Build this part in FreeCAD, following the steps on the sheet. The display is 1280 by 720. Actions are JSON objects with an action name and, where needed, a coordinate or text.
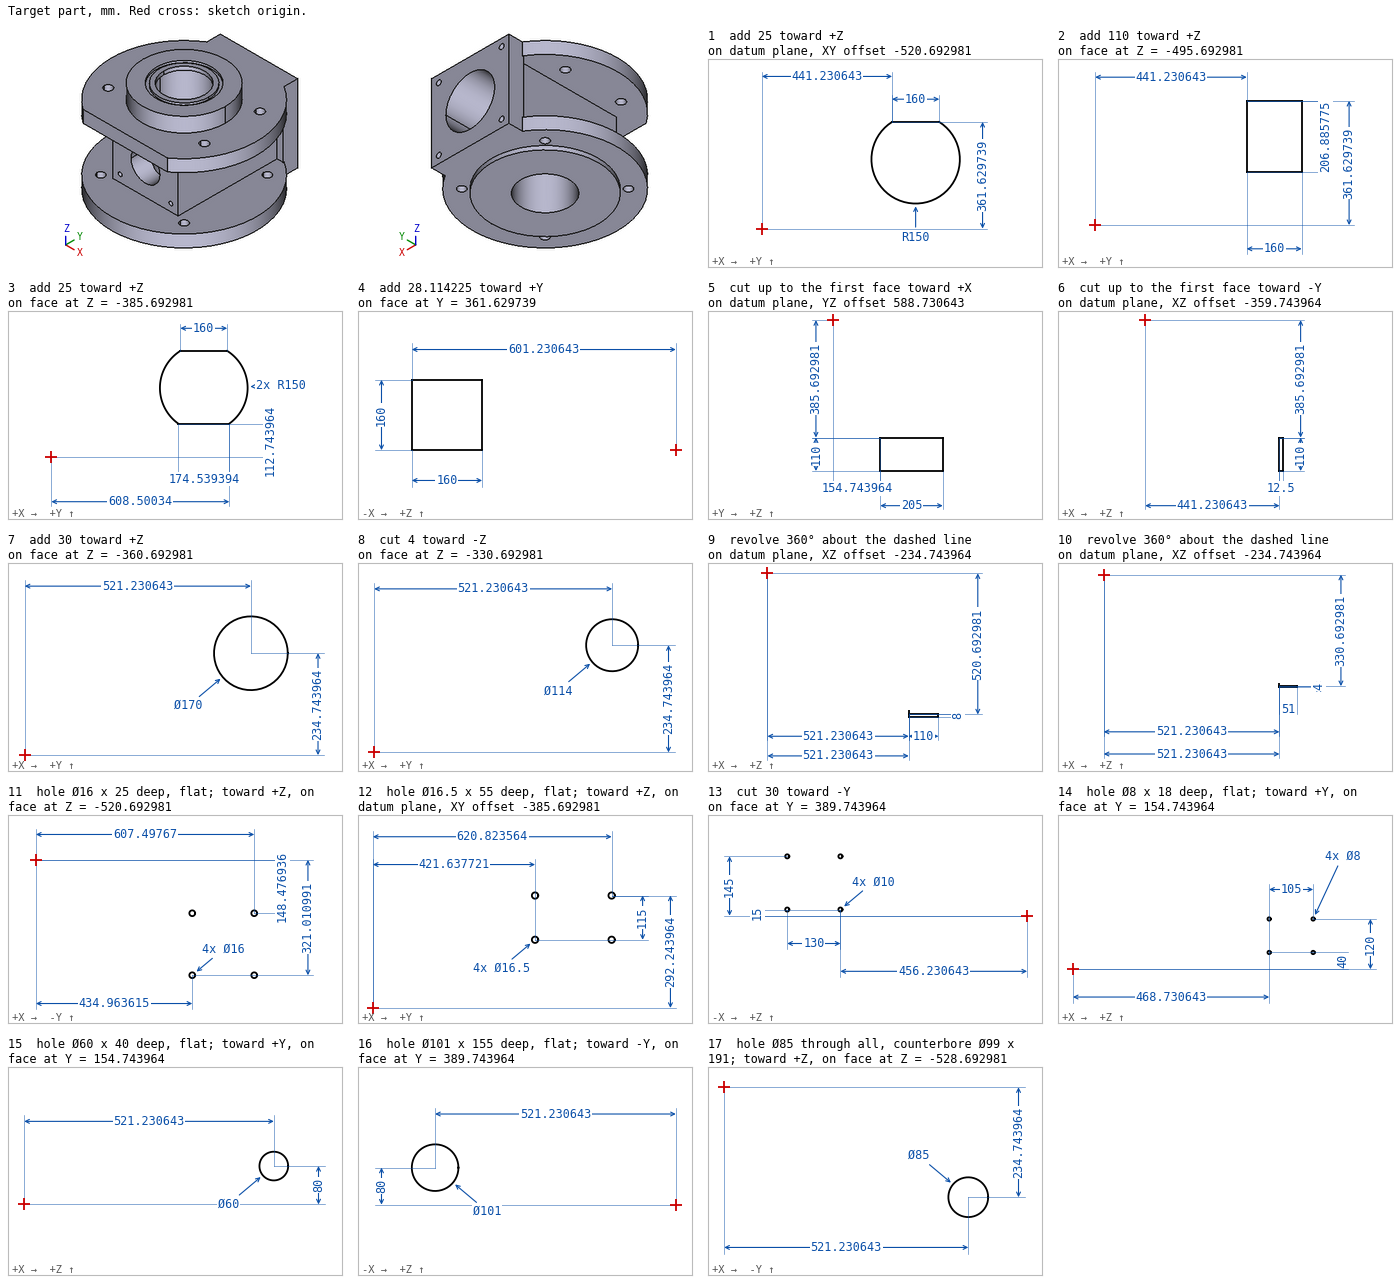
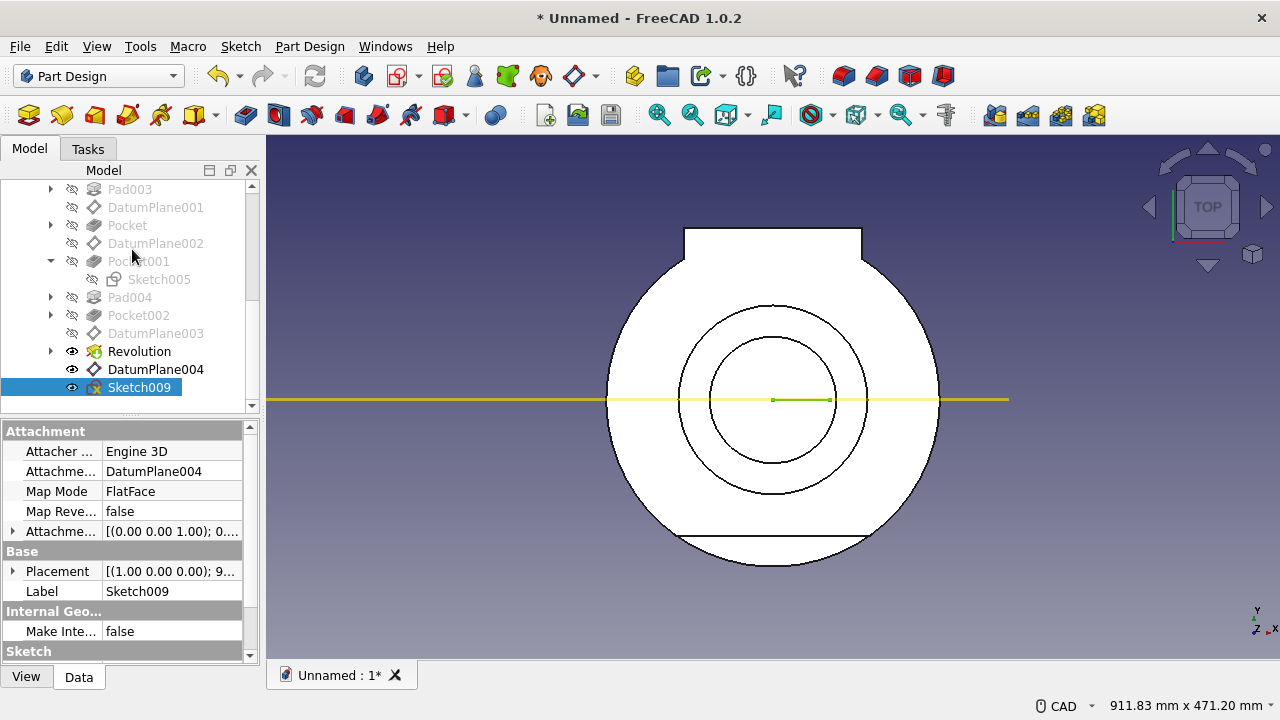
{"action": "left_click", "coordinate": [62, 116]}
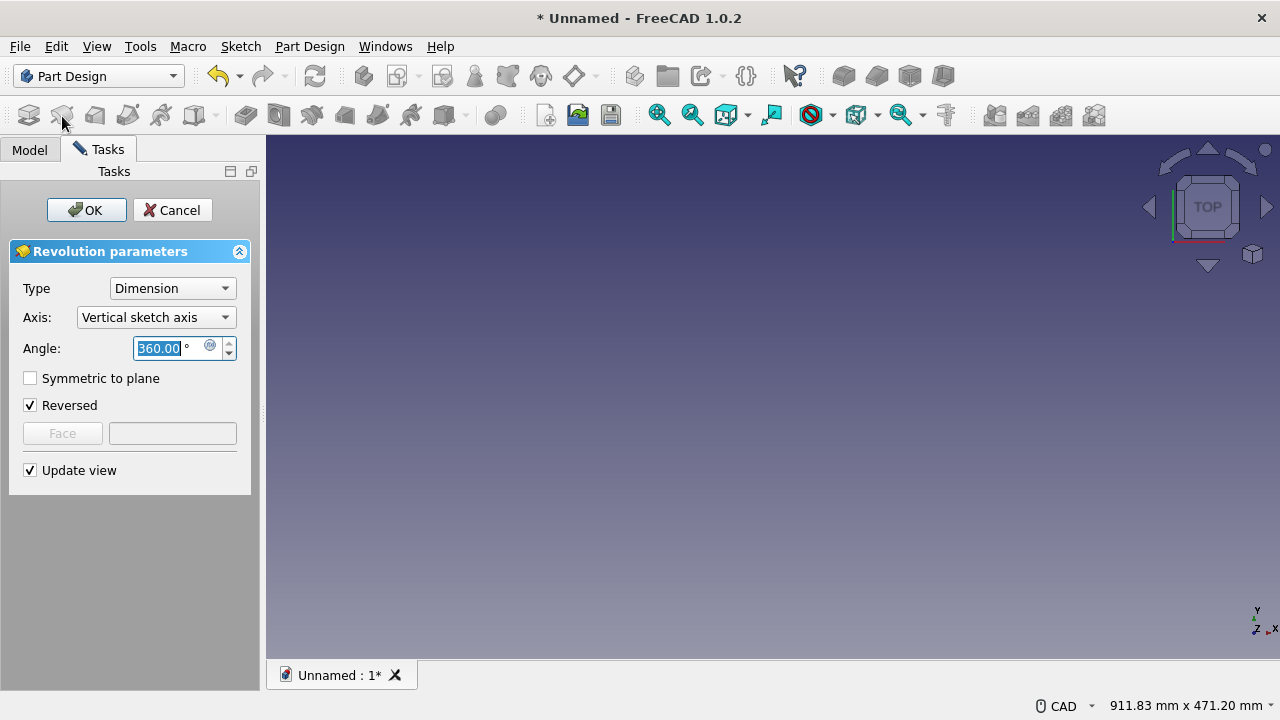
{"action": "left_click", "coordinate": [157, 318]}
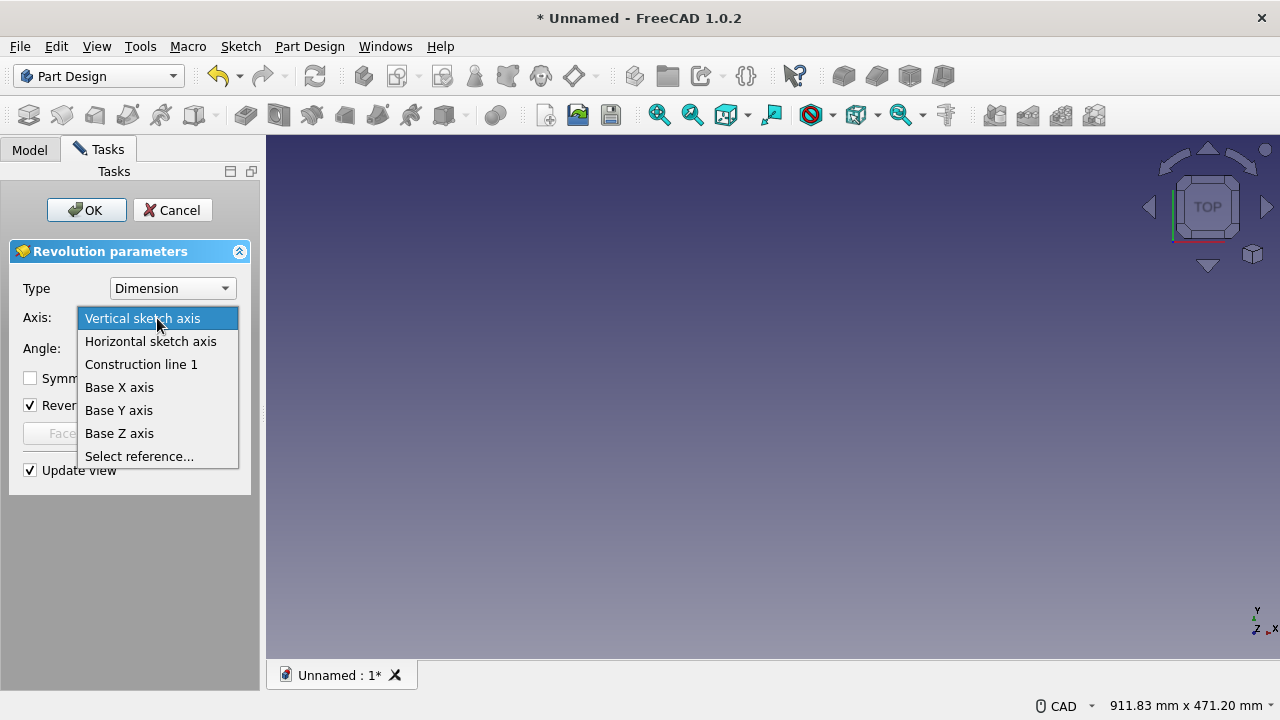
{"action": "left_click", "coordinate": [156, 364]}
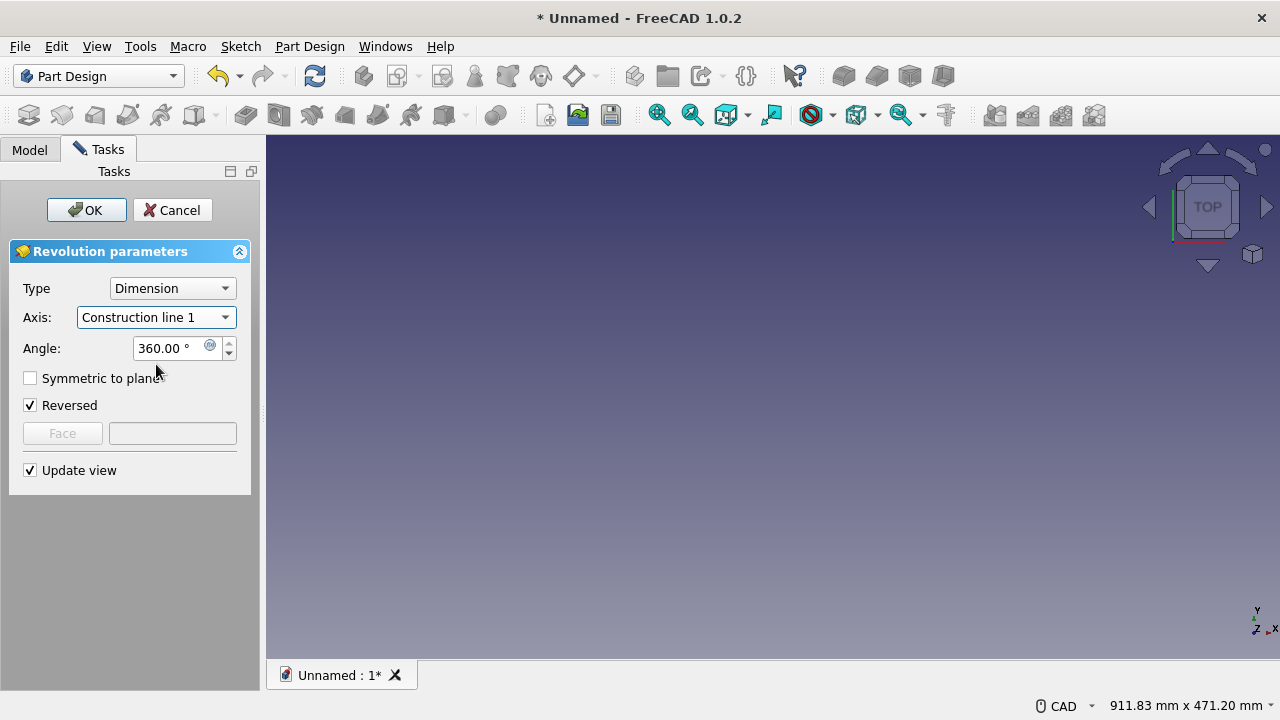
{"action": "left_click", "coordinate": [87, 210]}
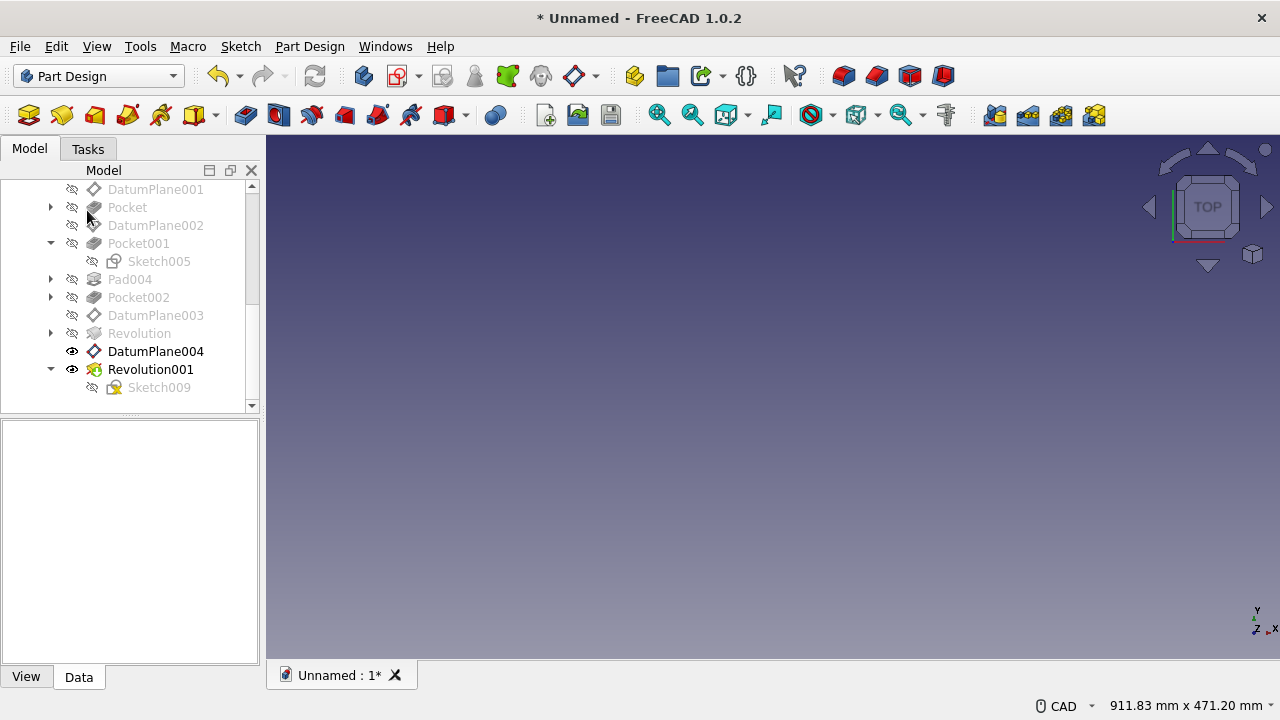
{"action": "left_click", "coordinate": [117, 351]}
{"action": "key", "text": "space"}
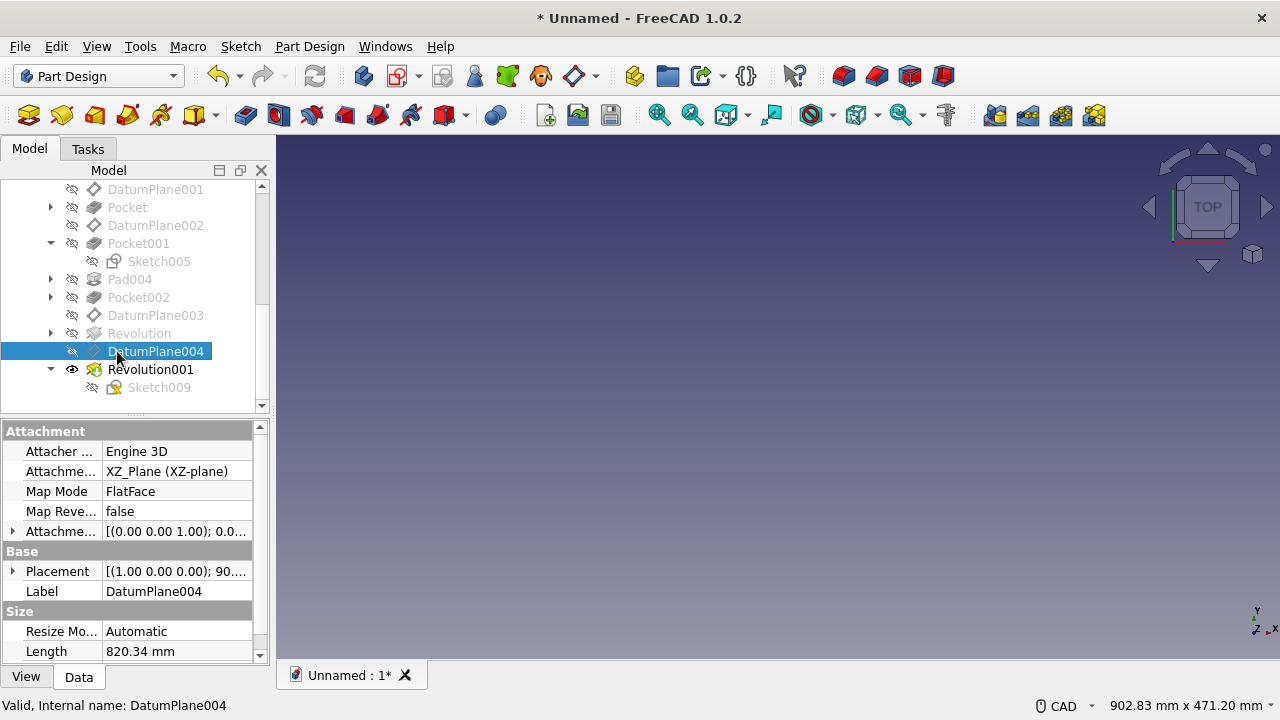
{"action": "left_click", "coordinate": [660, 116]}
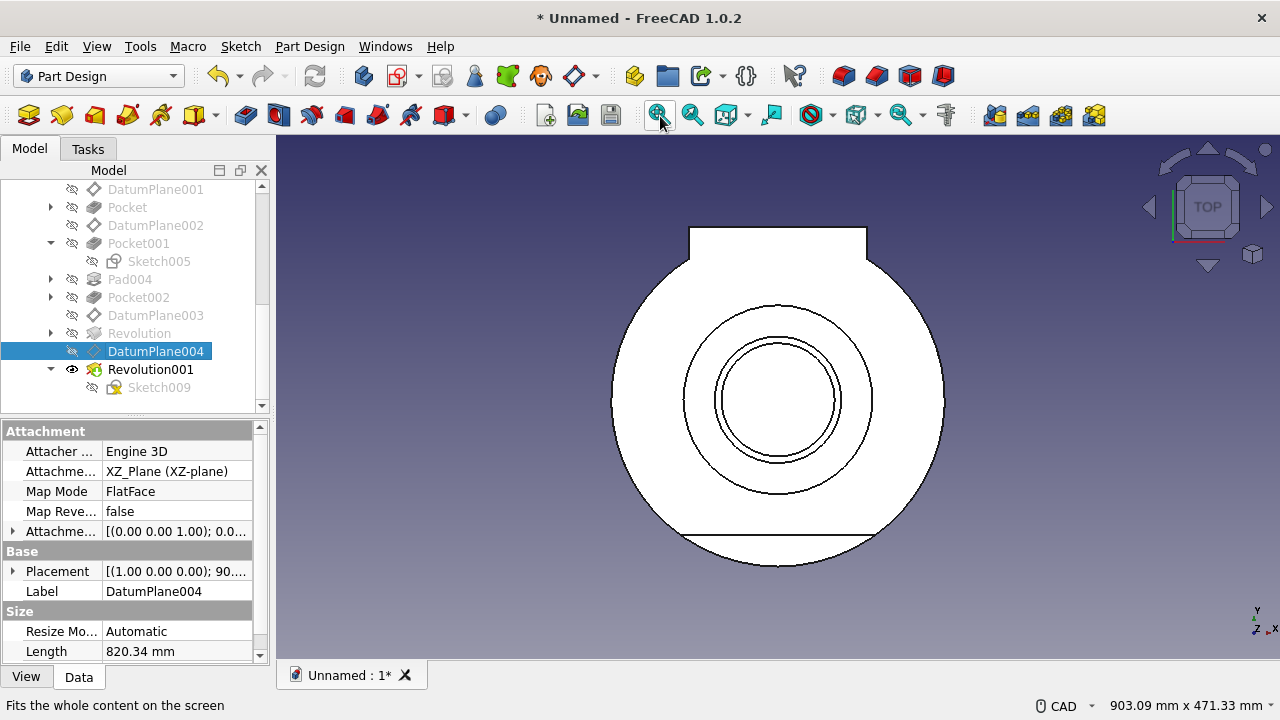
{"action": "key", "text": "5"}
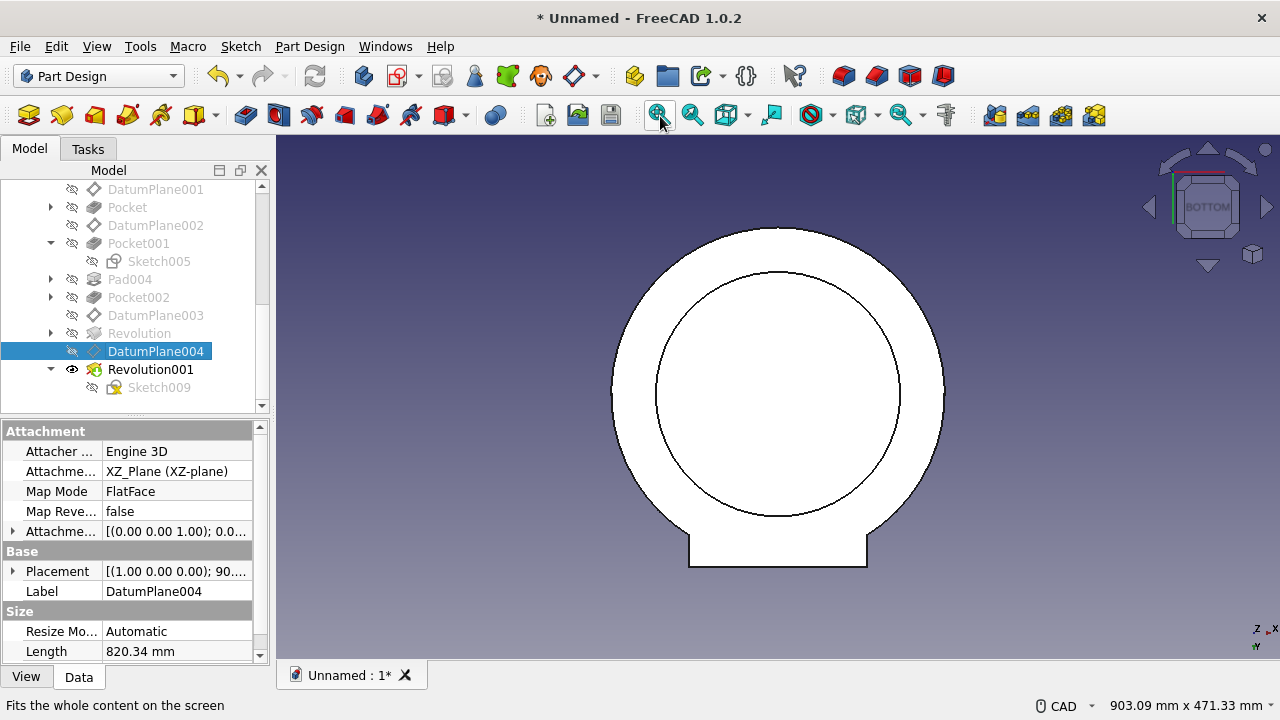
{"action": "left_click", "coordinate": [826, 541]}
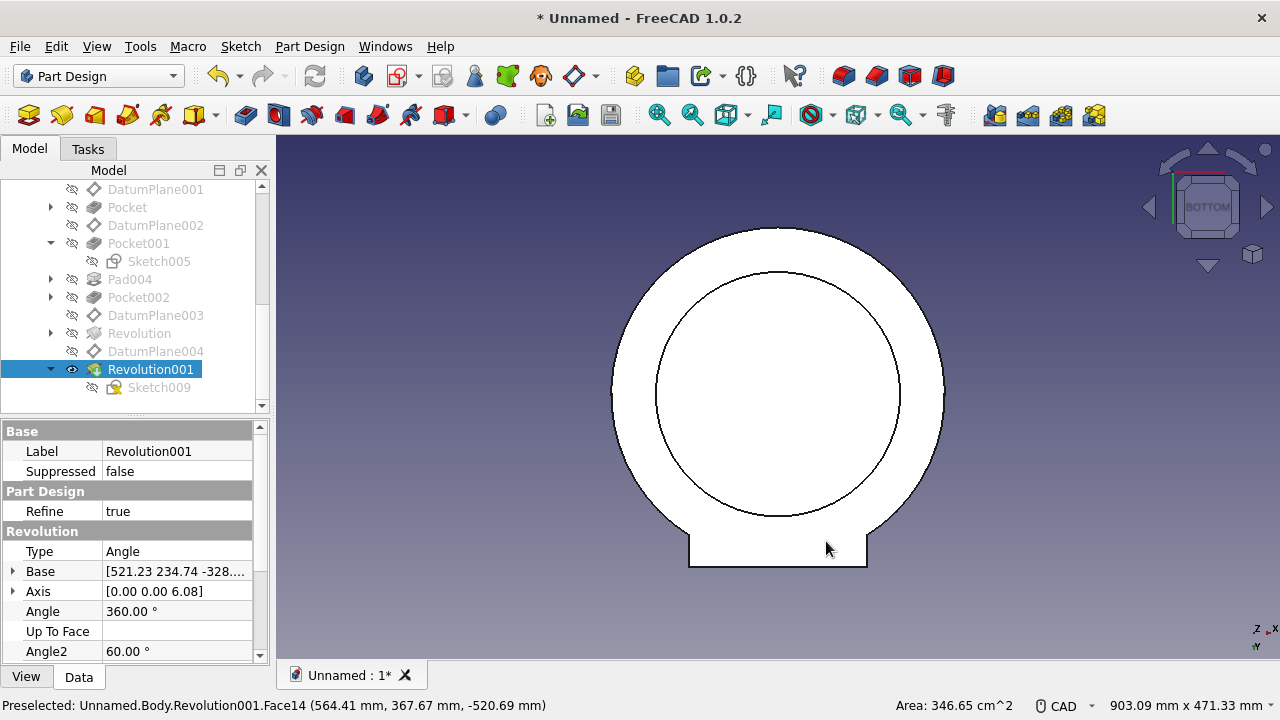
{"action": "left_click", "coordinate": [396, 76]}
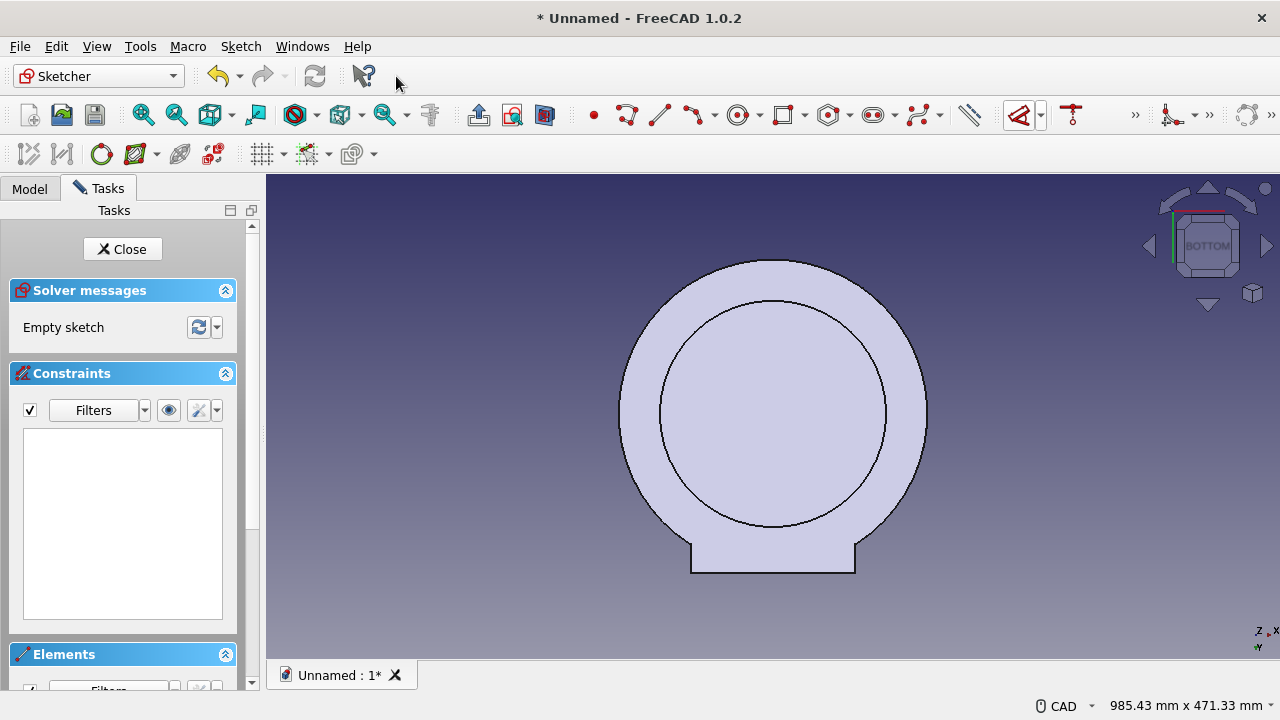
{"action": "scroll", "coordinate": [912, 409], "scroll_direction": "up", "scroll_amount": 2}